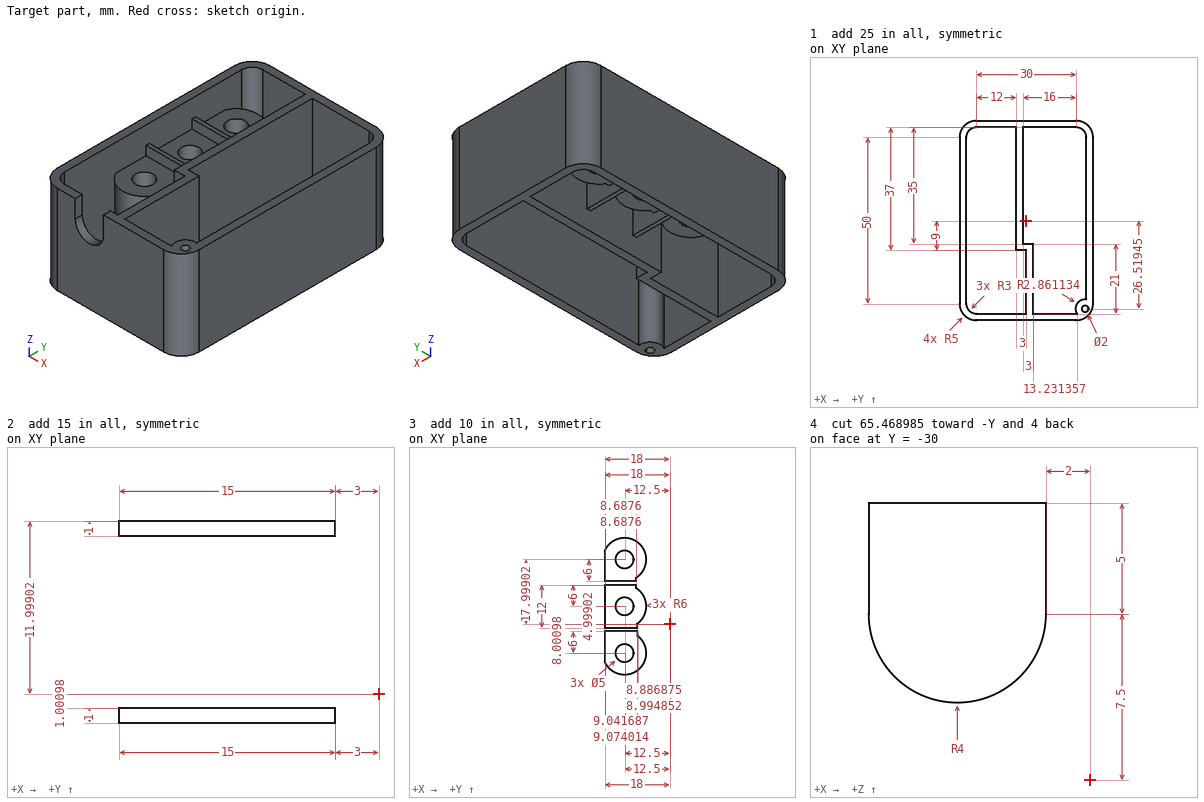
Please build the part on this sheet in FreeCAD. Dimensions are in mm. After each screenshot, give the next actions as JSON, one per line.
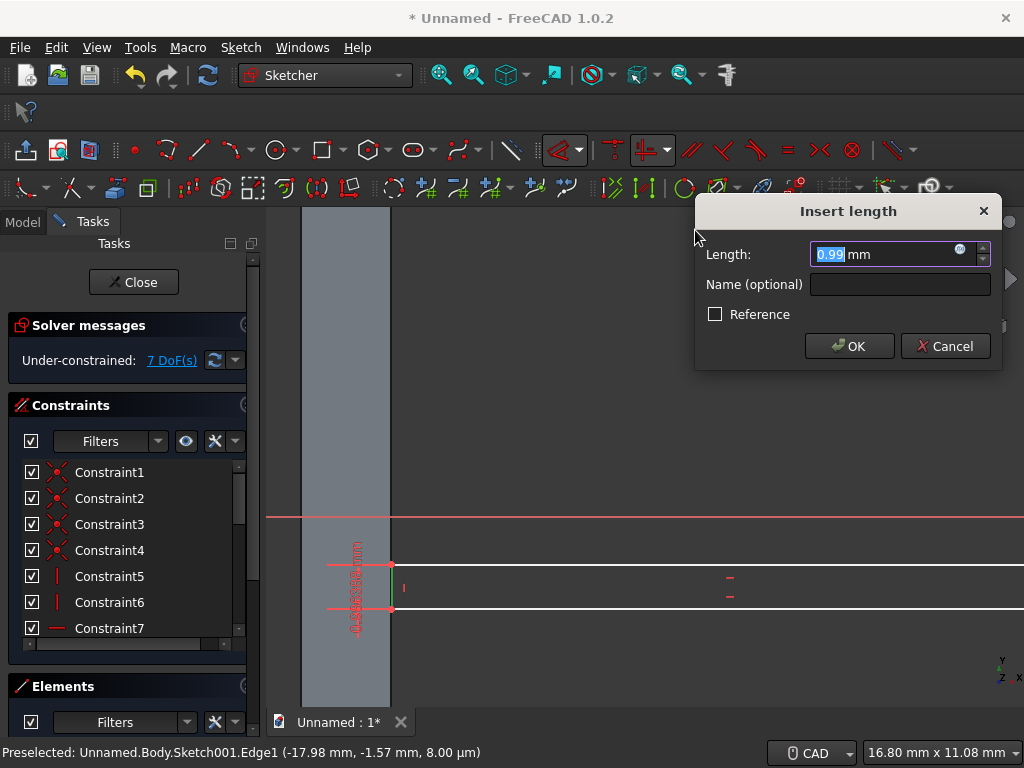
{"action": "type", "text": "1"}
{"action": "key", "text": "Return"}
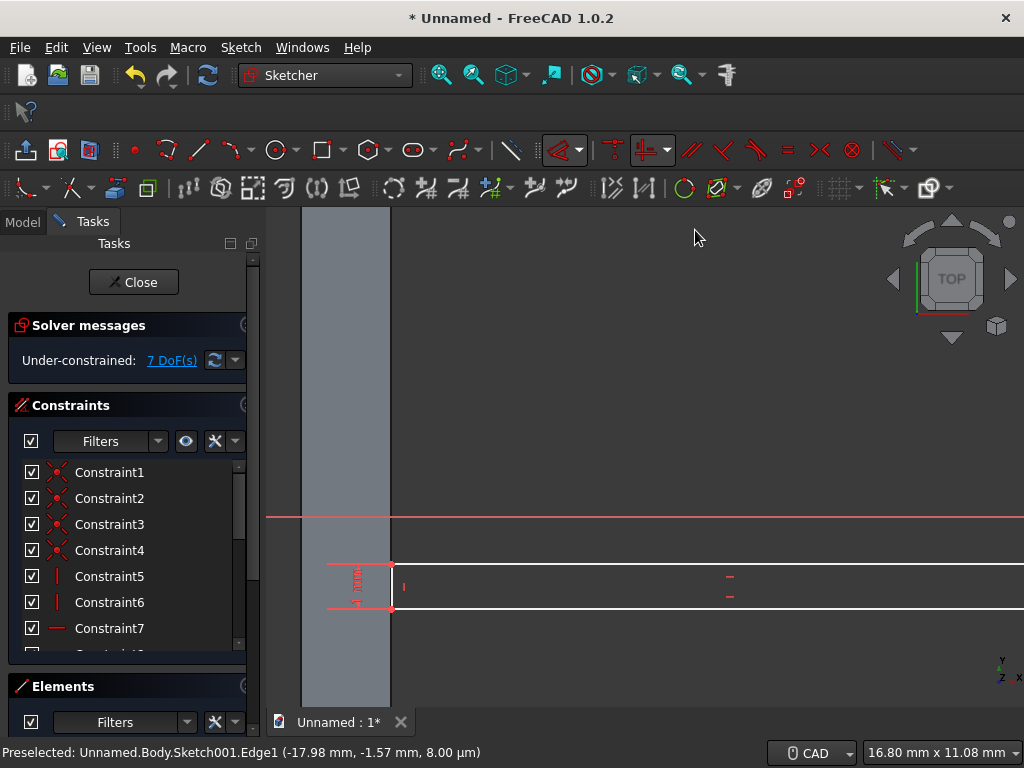
{"action": "scroll", "coordinate": [396, 592], "scroll_direction": "down", "scroll_amount": 4}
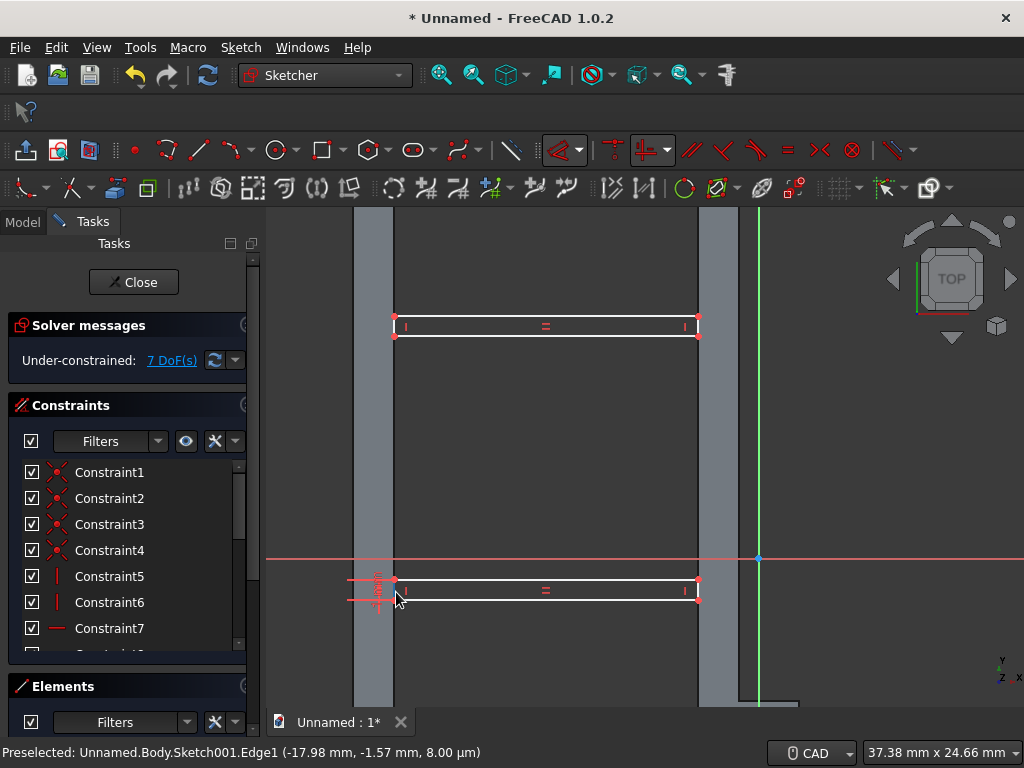
{"action": "scroll", "coordinate": [394, 322], "scroll_direction": "up", "scroll_amount": 5}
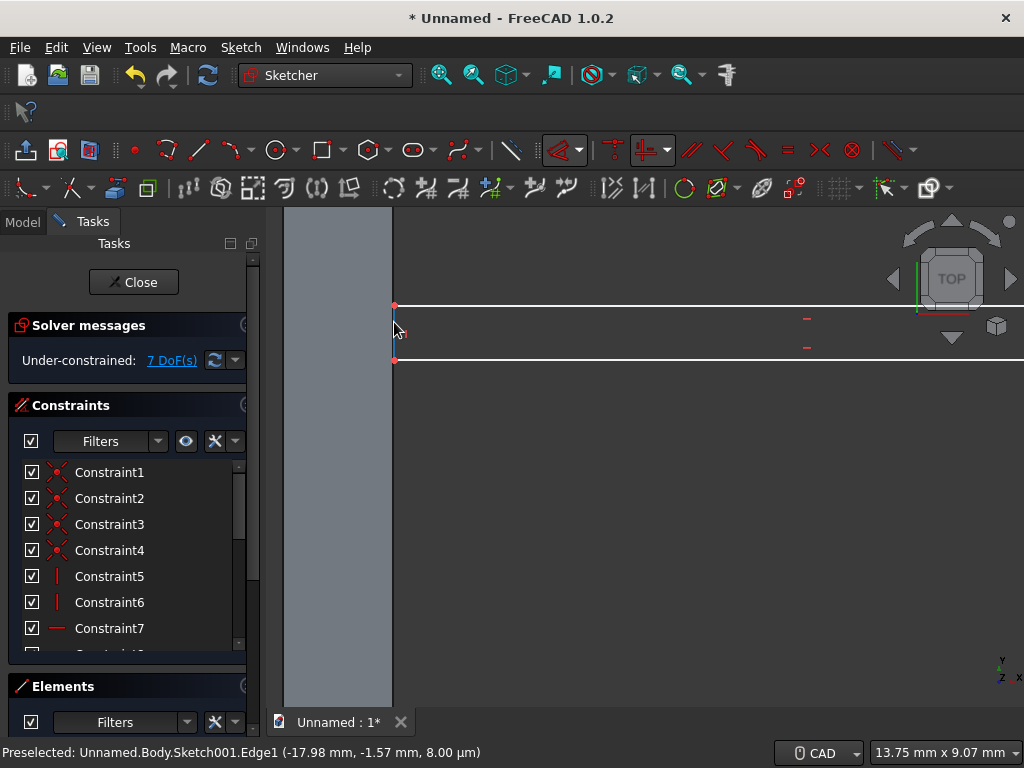
{"action": "left_click", "coordinate": [394, 322]}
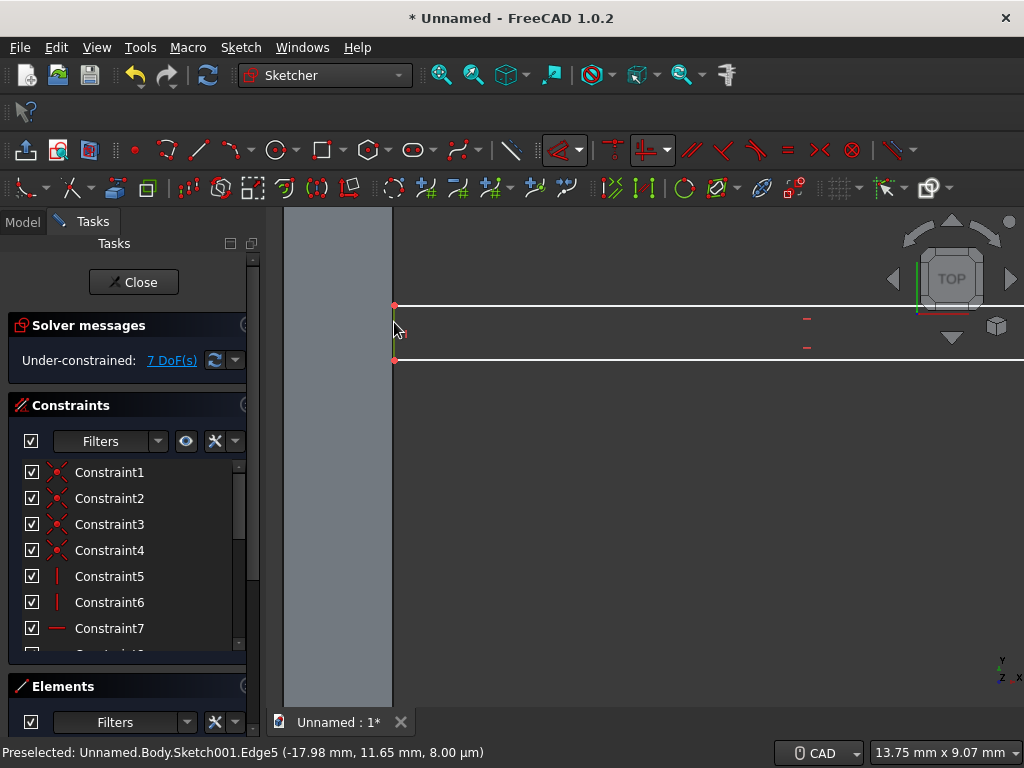
{"action": "left_click", "coordinate": [582, 150]}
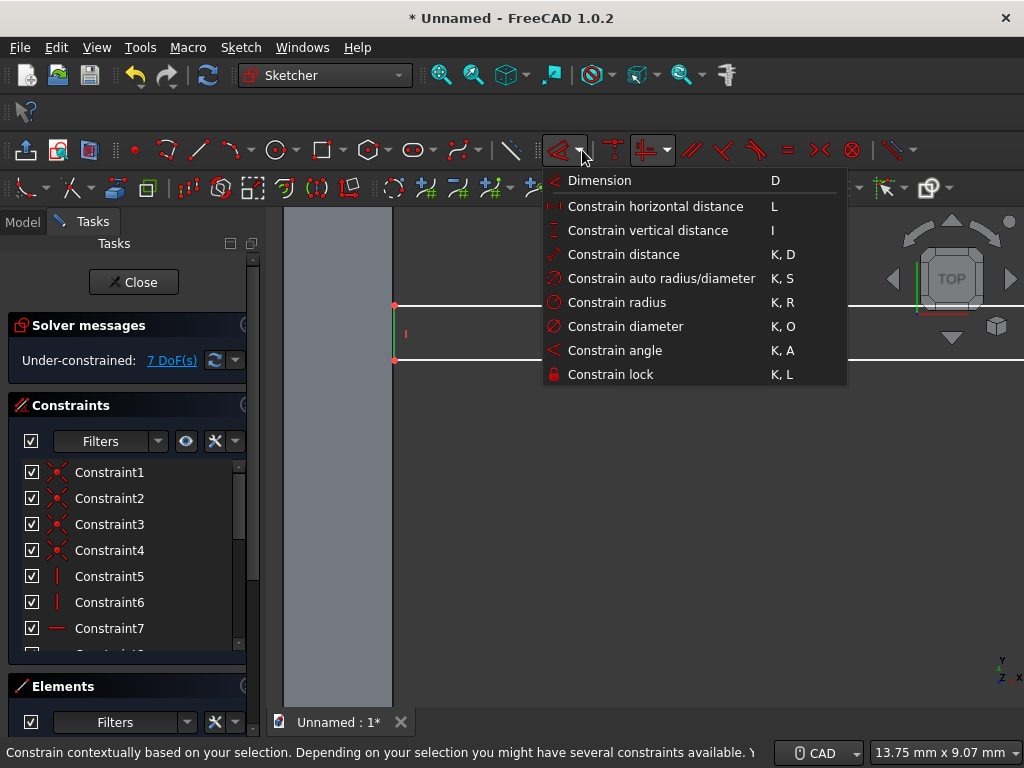
{"action": "left_click", "coordinate": [695, 230]}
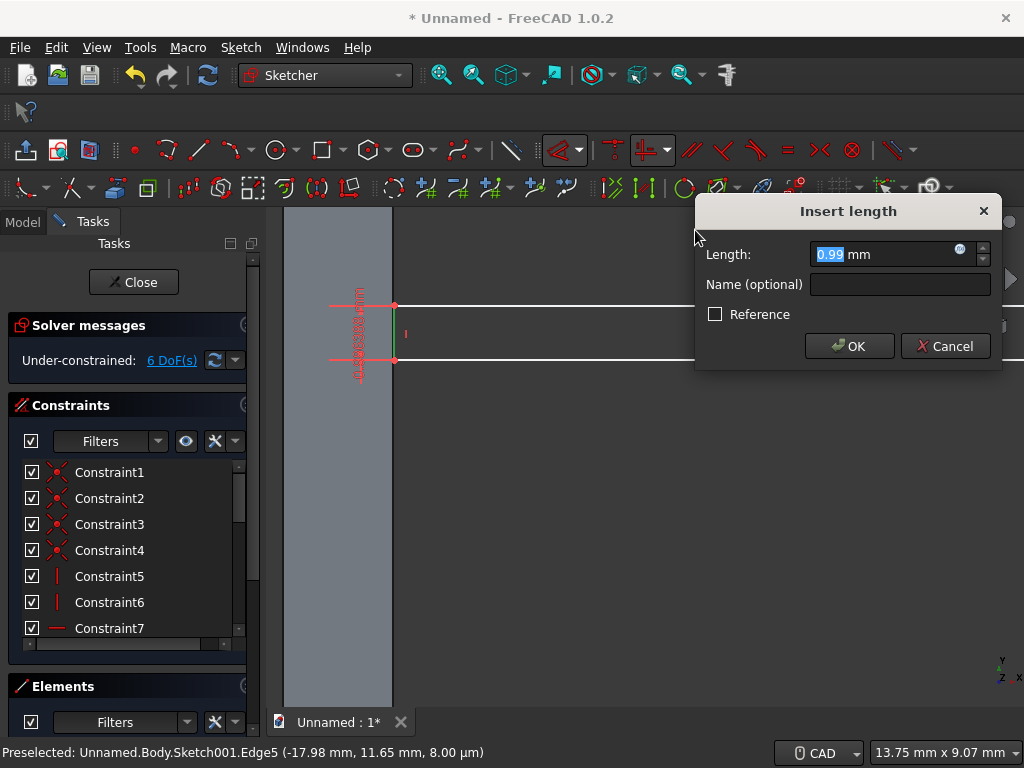
{"action": "type", "text": "1"}
{"action": "key", "text": "Return"}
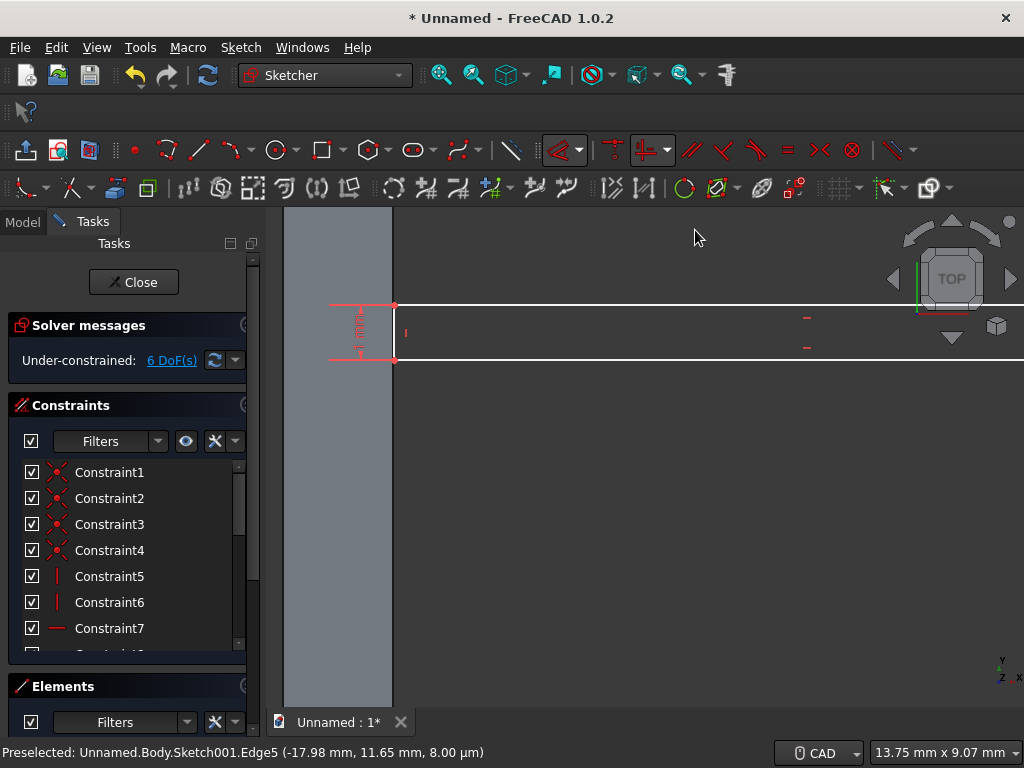
{"action": "scroll", "coordinate": [394, 322], "scroll_direction": "down", "scroll_amount": 5}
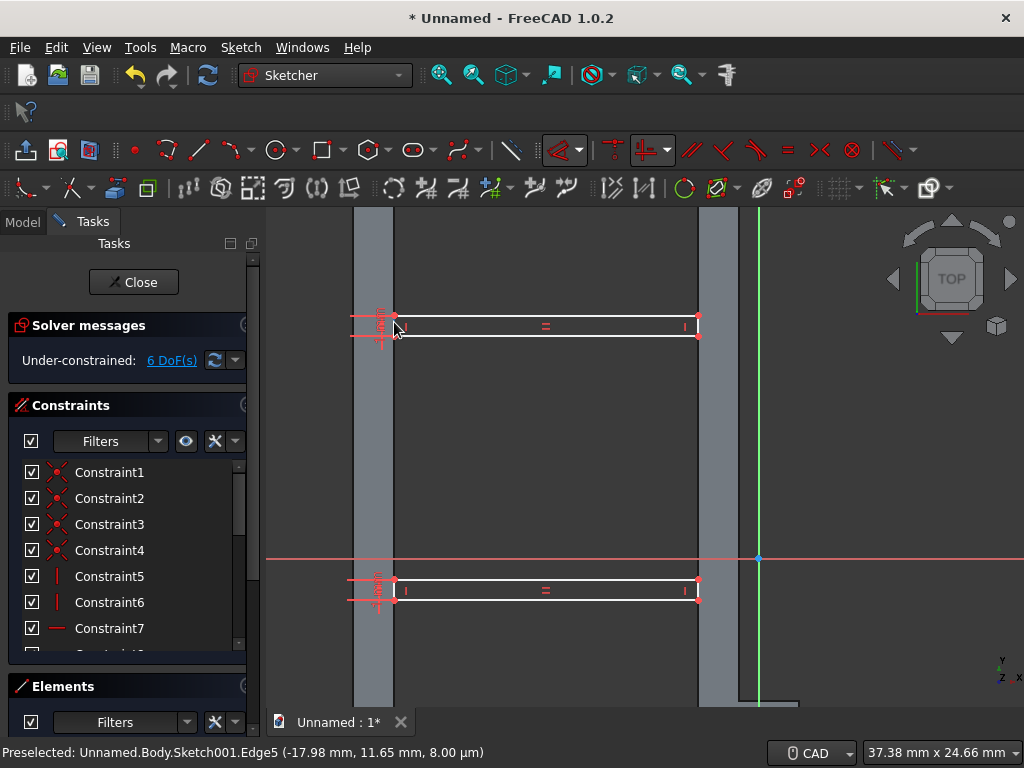
{"action": "left_click", "coordinate": [485, 600]}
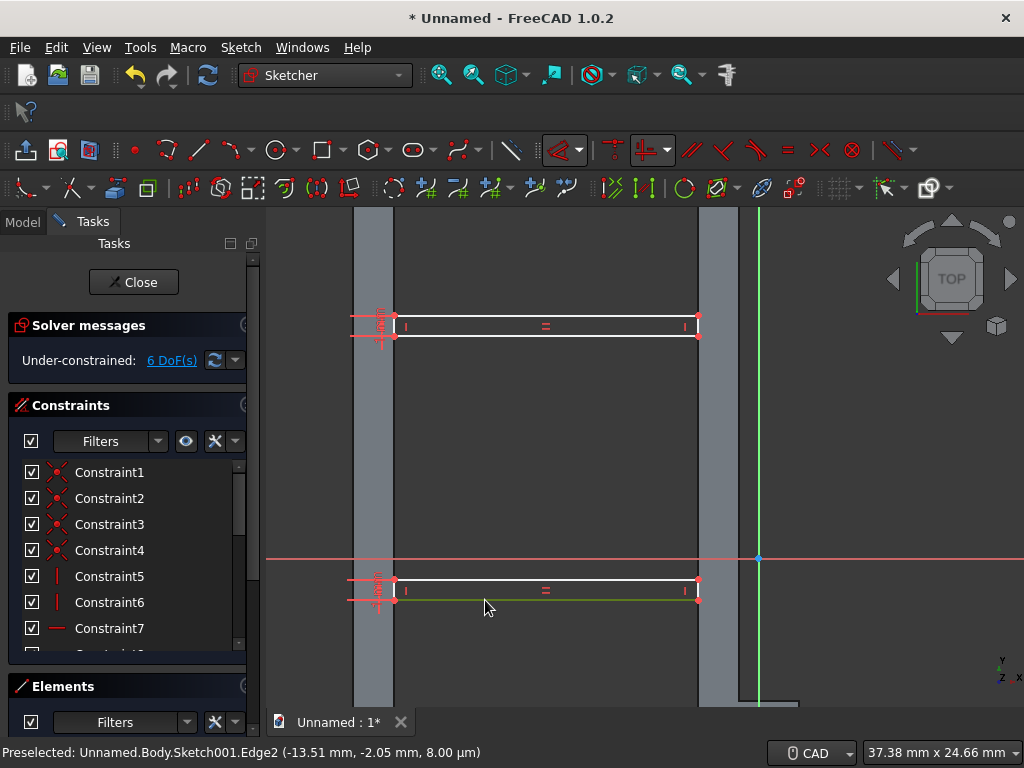
{"action": "left_click", "coordinate": [582, 150]}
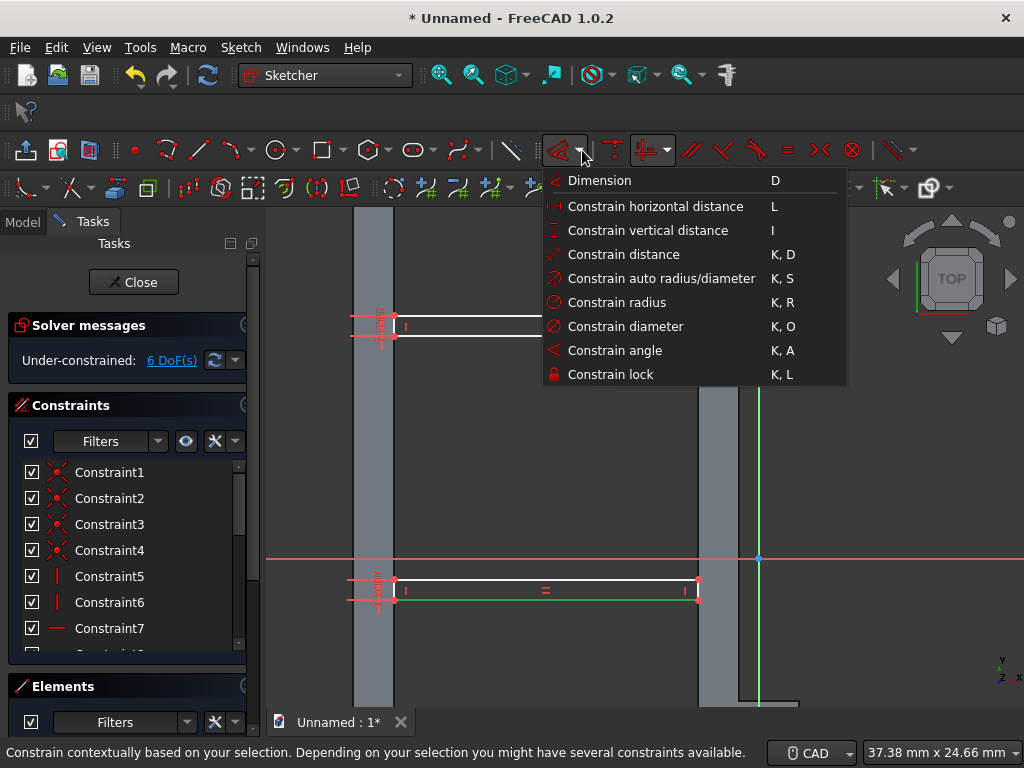
{"action": "left_click", "coordinate": [695, 206]}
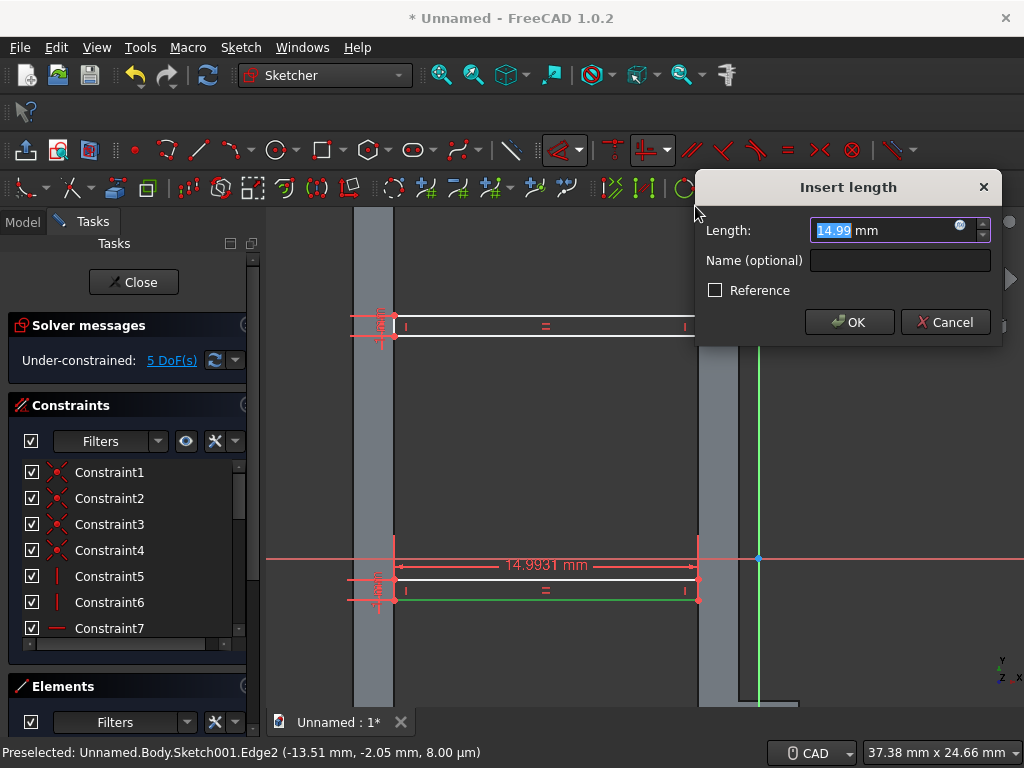
{"action": "type", "text": "15"}
{"action": "key", "text": "Return"}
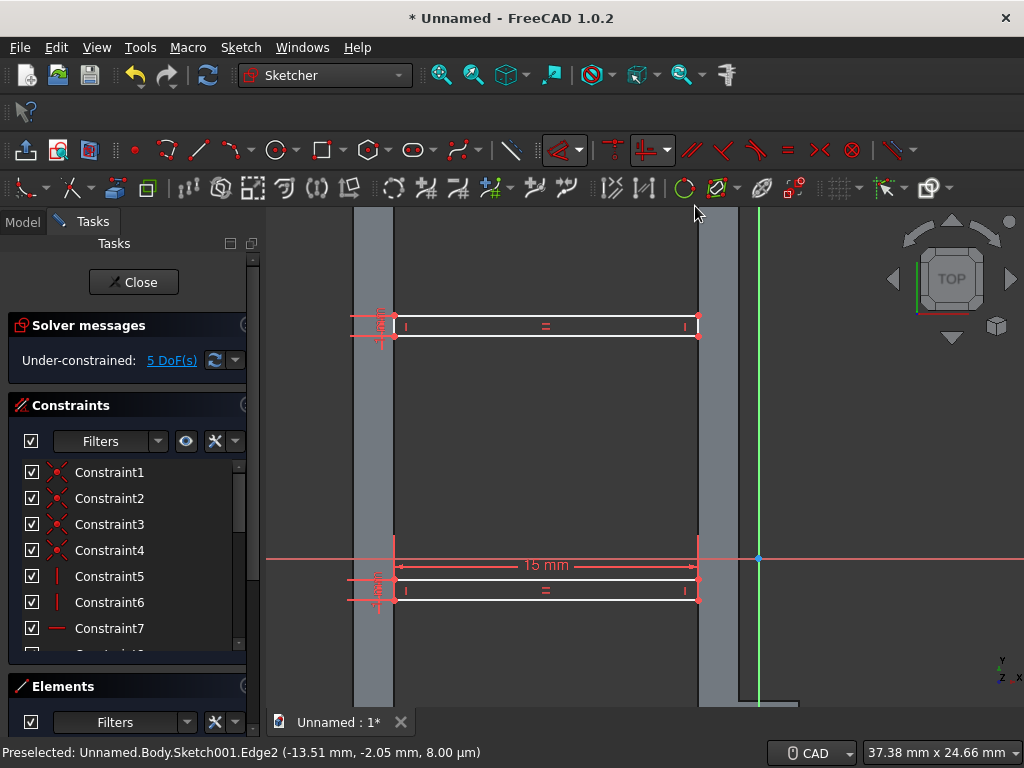
{"action": "left_click", "coordinate": [485, 336]}